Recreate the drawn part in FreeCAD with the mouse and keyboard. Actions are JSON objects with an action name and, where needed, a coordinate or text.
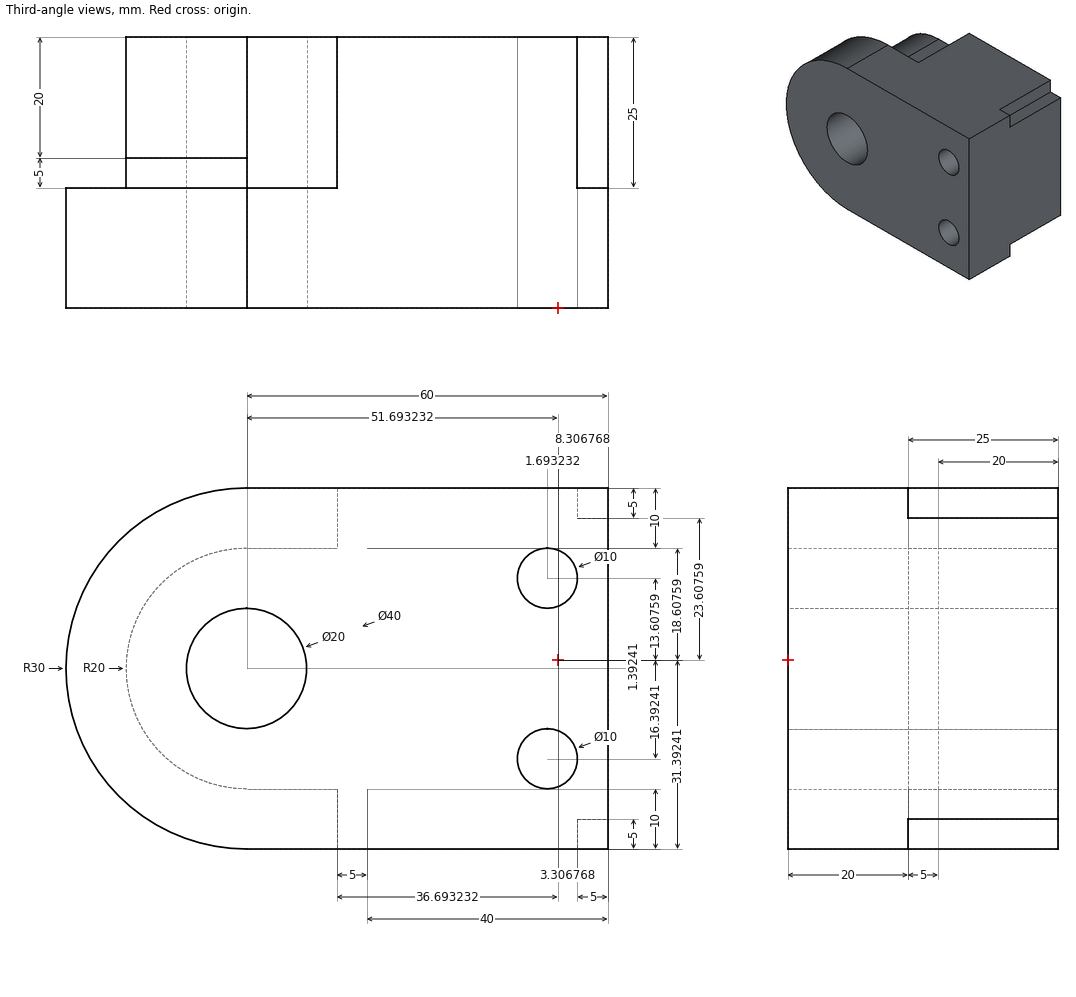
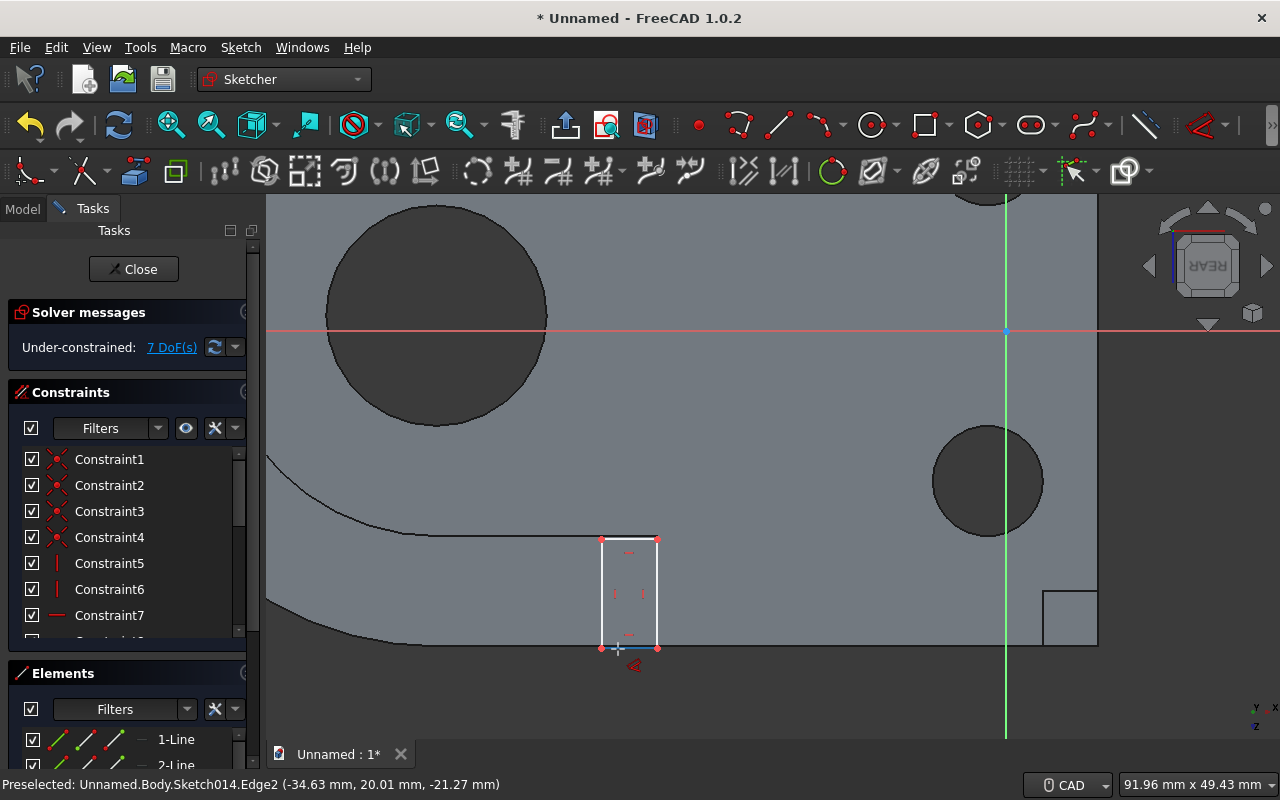
{"action": "left_click", "coordinate": [619, 648]}
{"action": "left_click", "coordinate": [630, 682]}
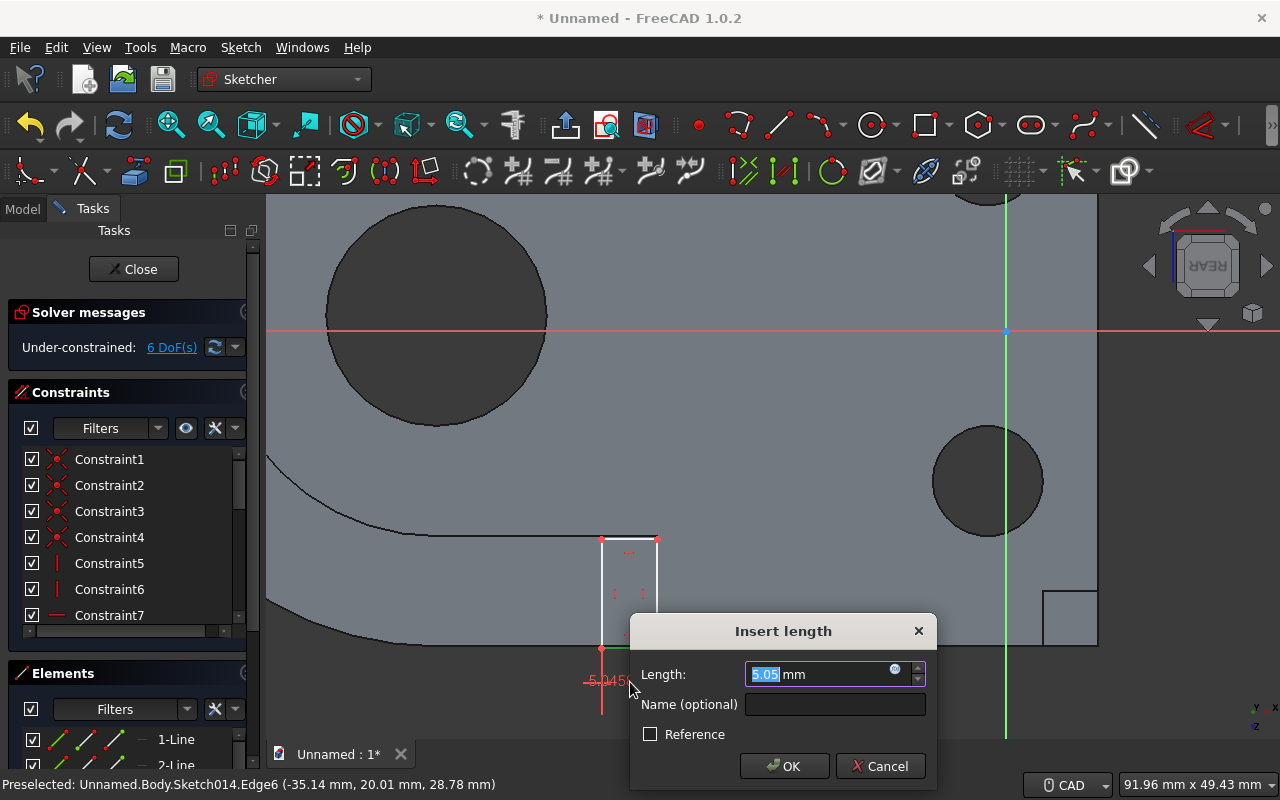
{"action": "type", "text": "5"}
{"action": "key", "text": "Return"}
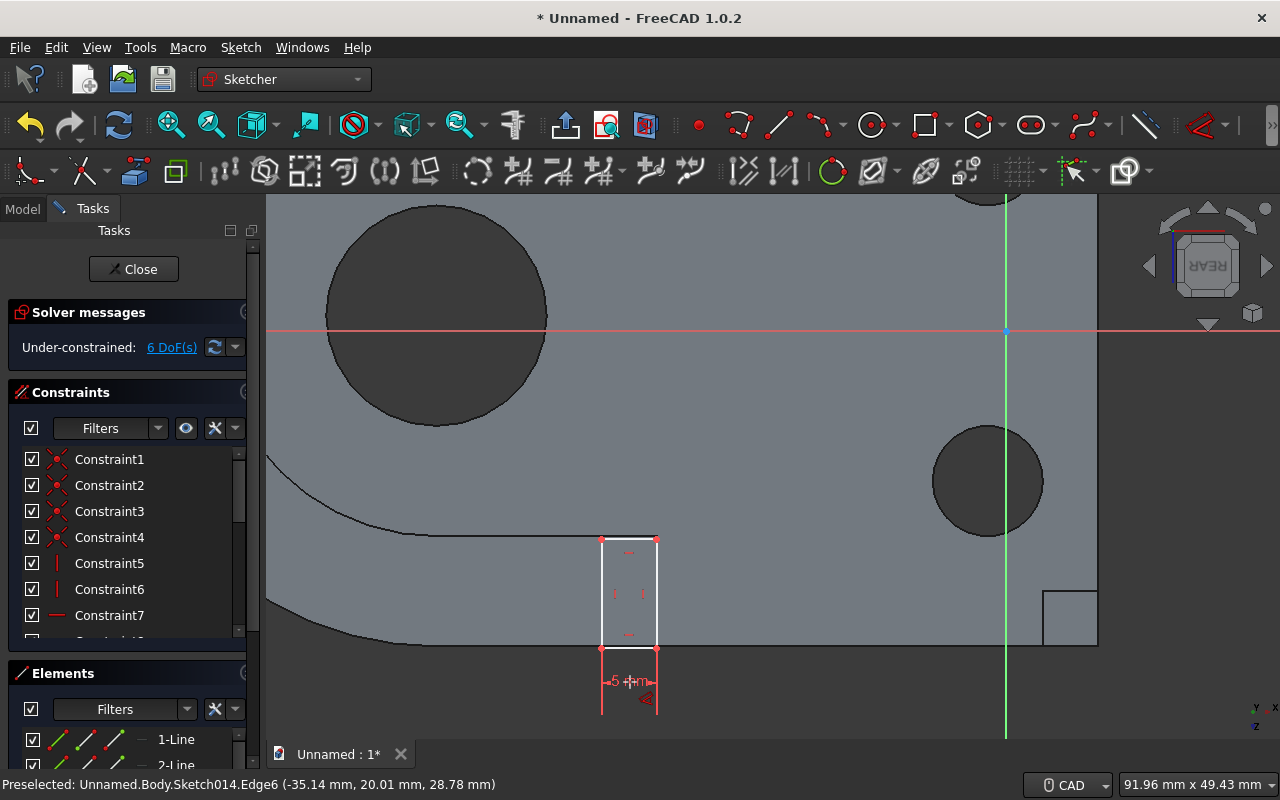
{"action": "scroll", "coordinate": [583, 650], "scroll_direction": "down", "scroll_amount": 3}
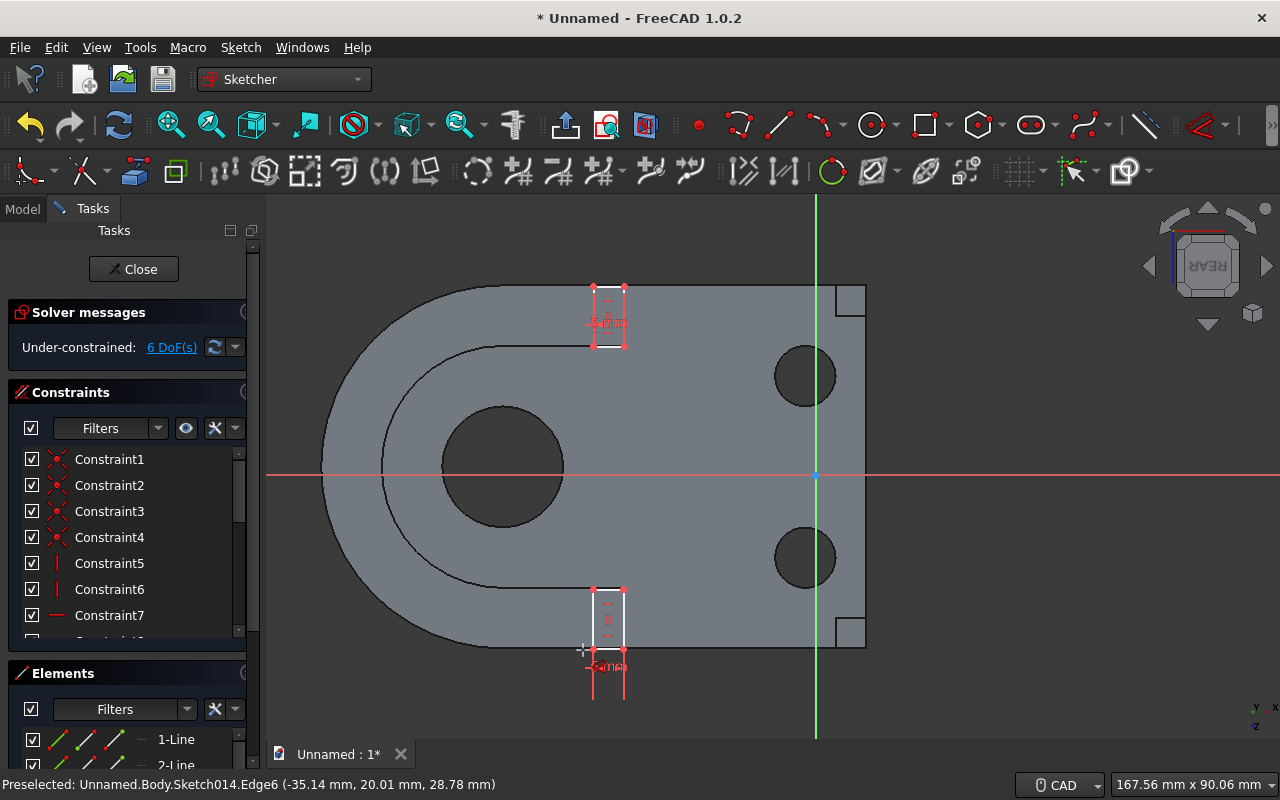
{"action": "left_click", "coordinate": [594, 305]}
{"action": "left_click", "coordinate": [560, 303]}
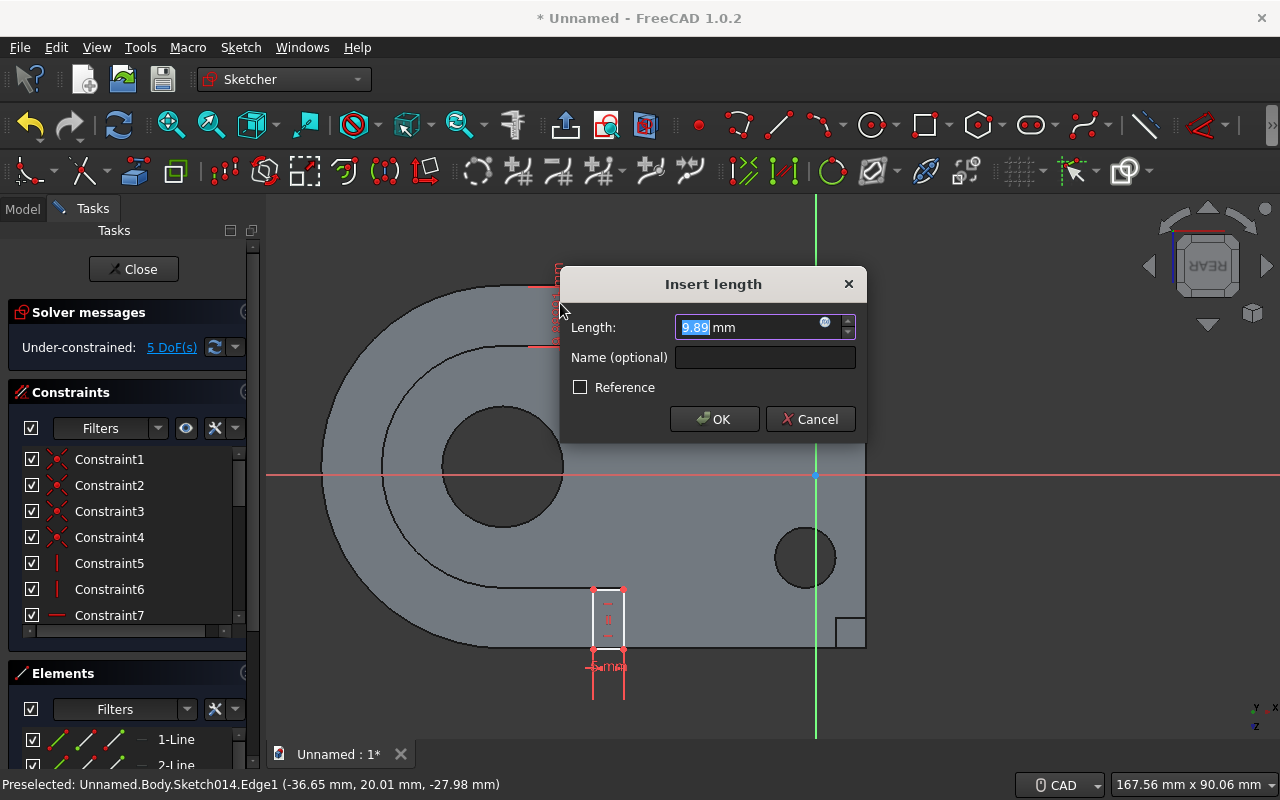
{"action": "type", "text": "10"}
{"action": "key", "text": "Return"}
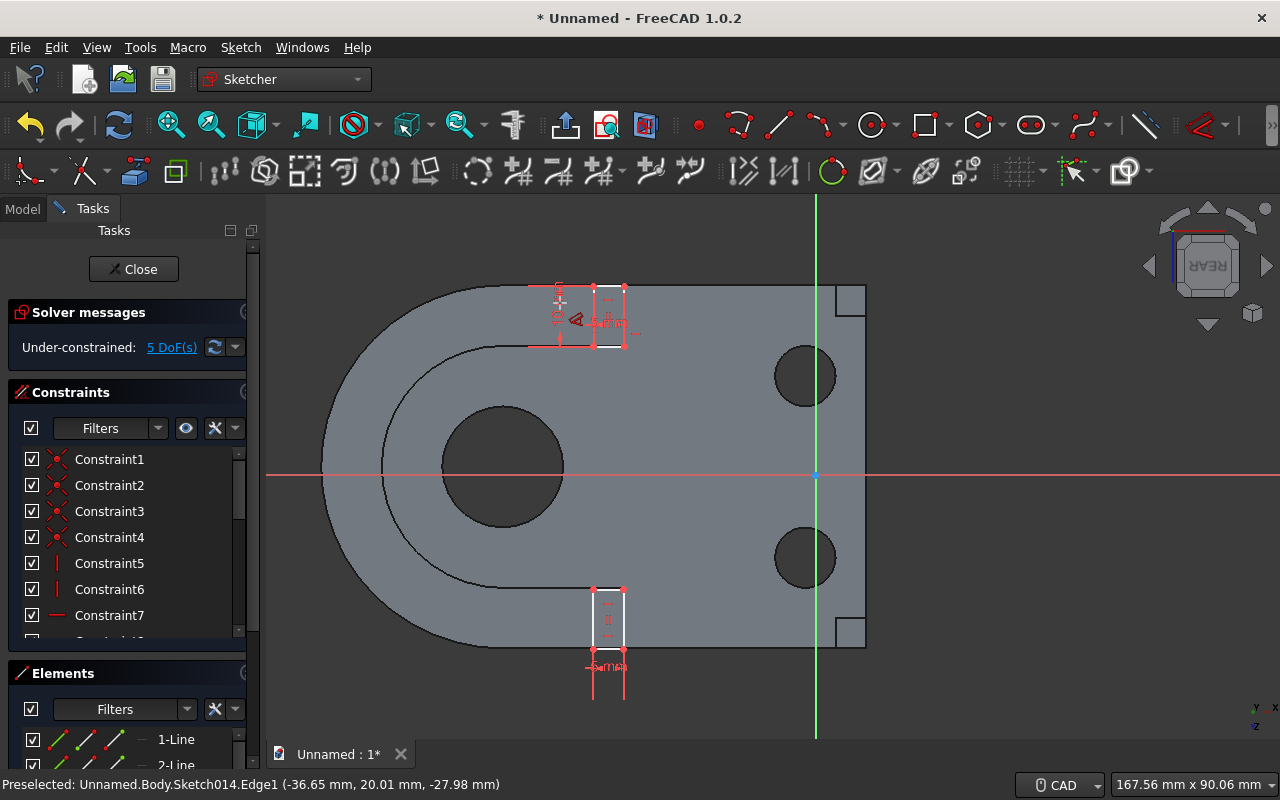
{"action": "left_click", "coordinate": [593, 608]}
{"action": "left_click", "coordinate": [559, 620]}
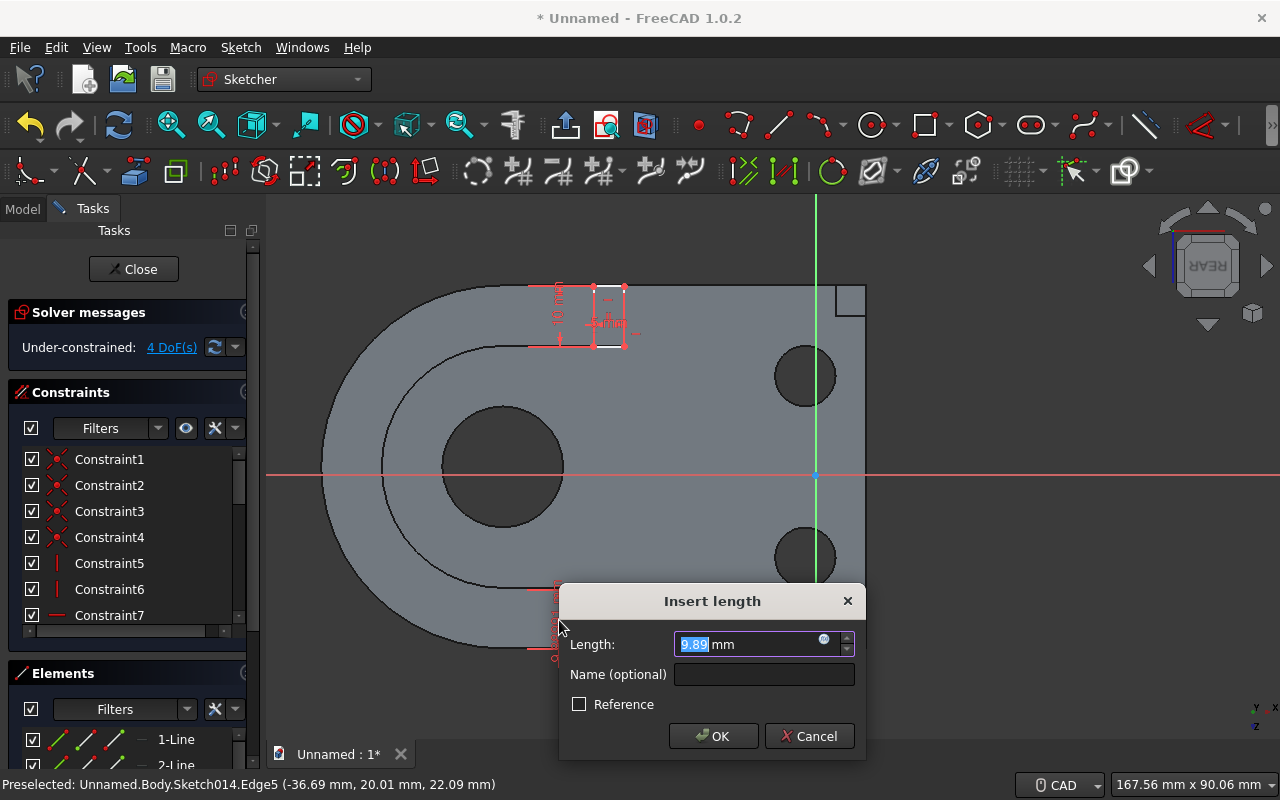
{"action": "type", "text": "10"}
{"action": "key", "text": "Return"}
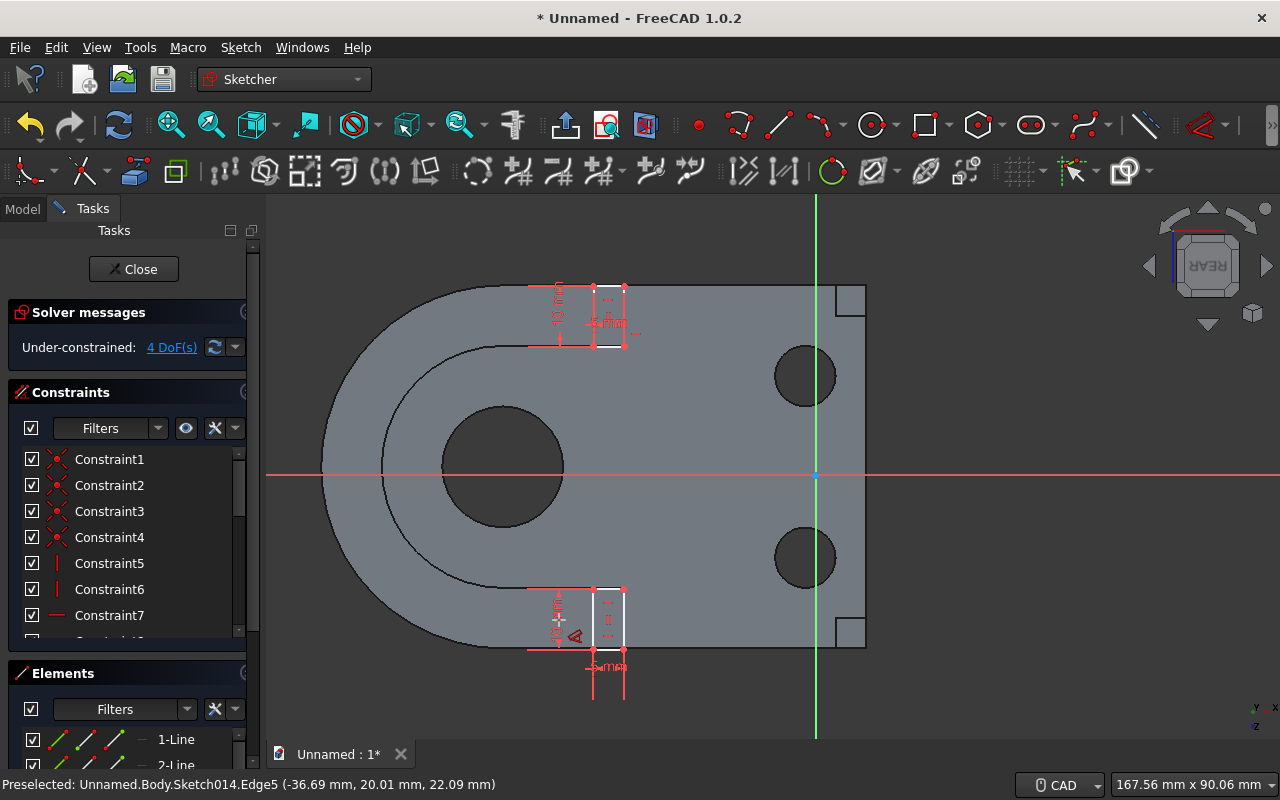
{"action": "left_click", "coordinate": [594, 286]}
{"action": "left_click", "coordinate": [850, 381]}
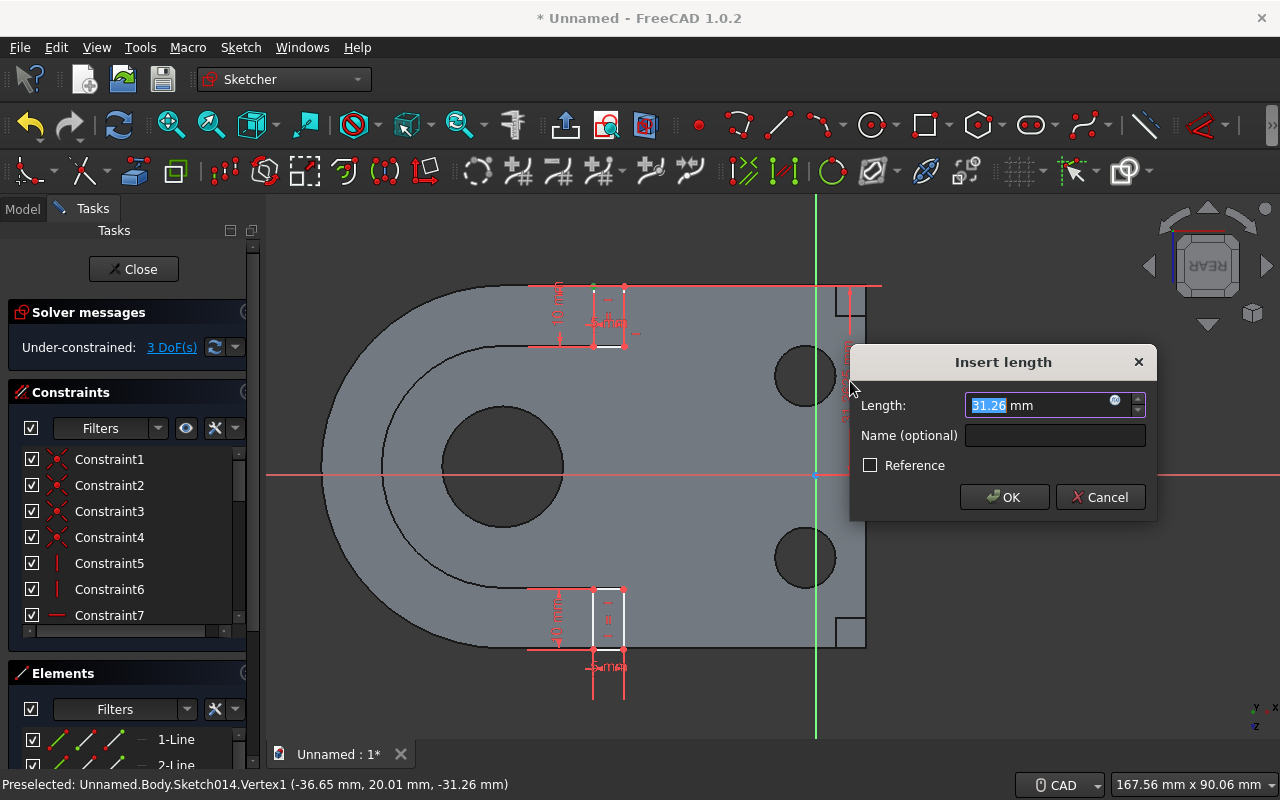
{"action": "type", "text": "31.39241"}
{"action": "key", "text": "Return"}